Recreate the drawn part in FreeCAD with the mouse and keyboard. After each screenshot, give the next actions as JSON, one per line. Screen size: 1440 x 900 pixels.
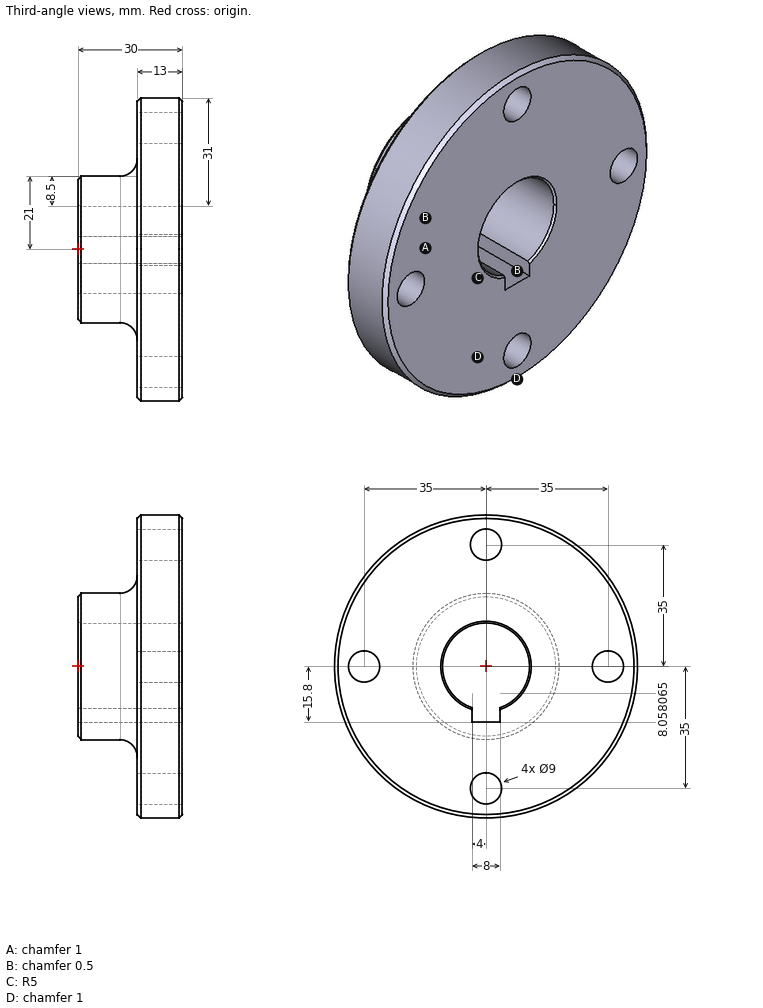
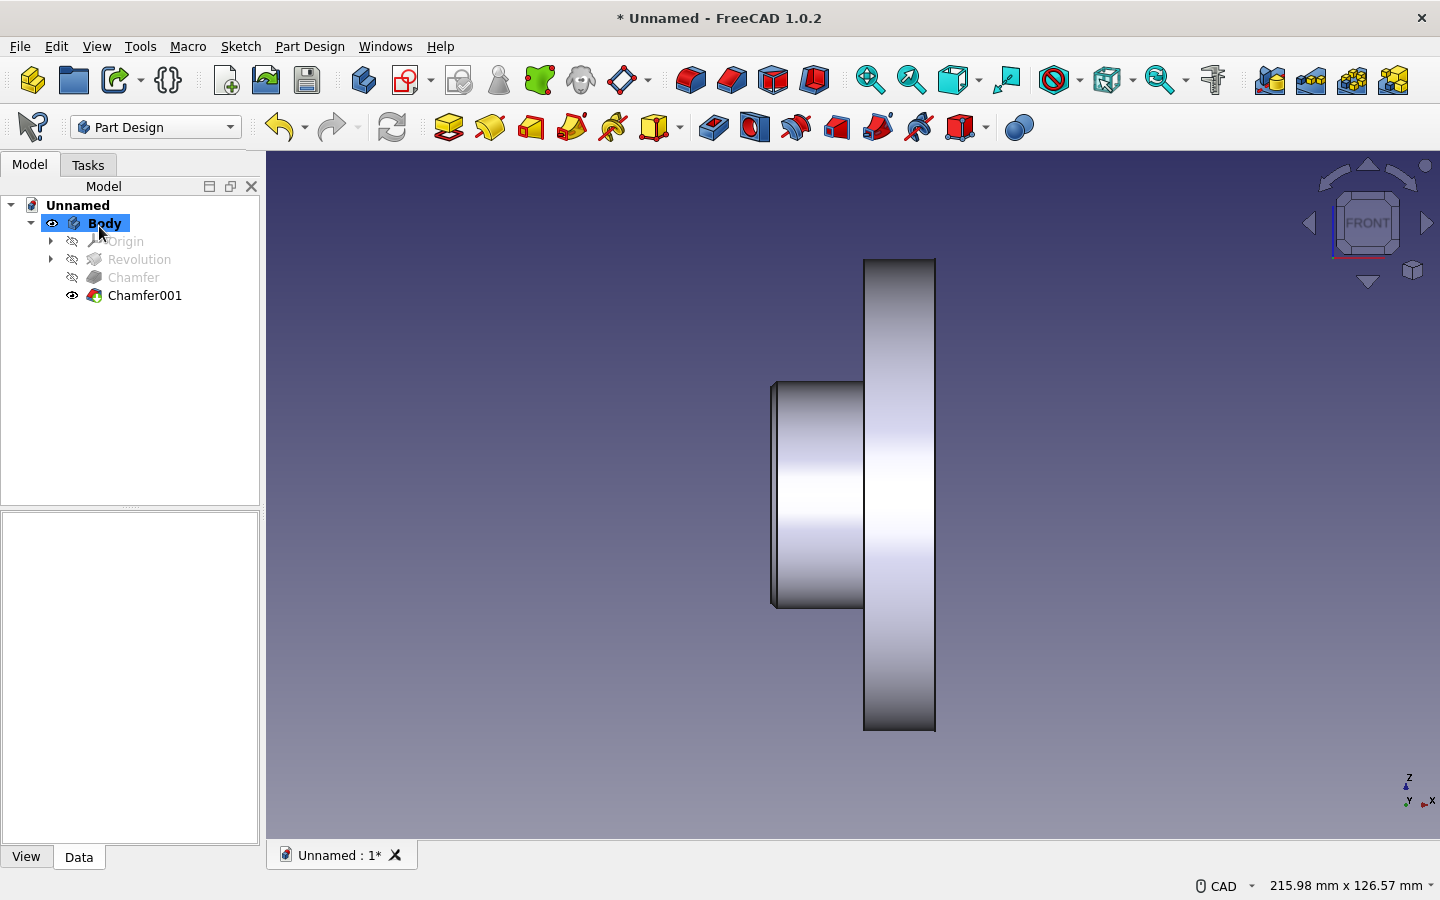
{"action": "key", "text": "3"}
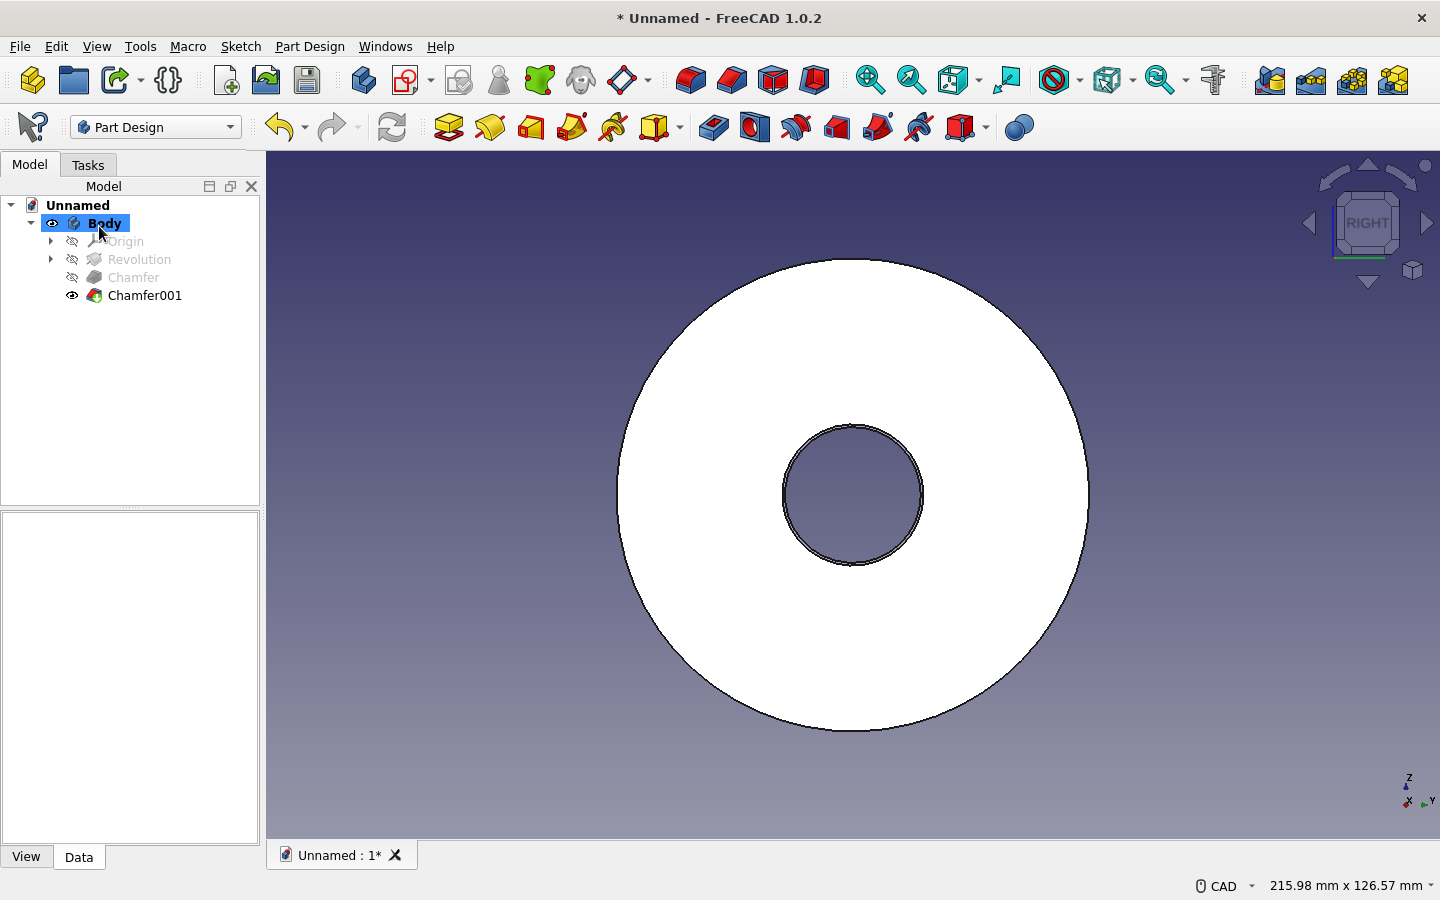
{"action": "key", "text": "5"}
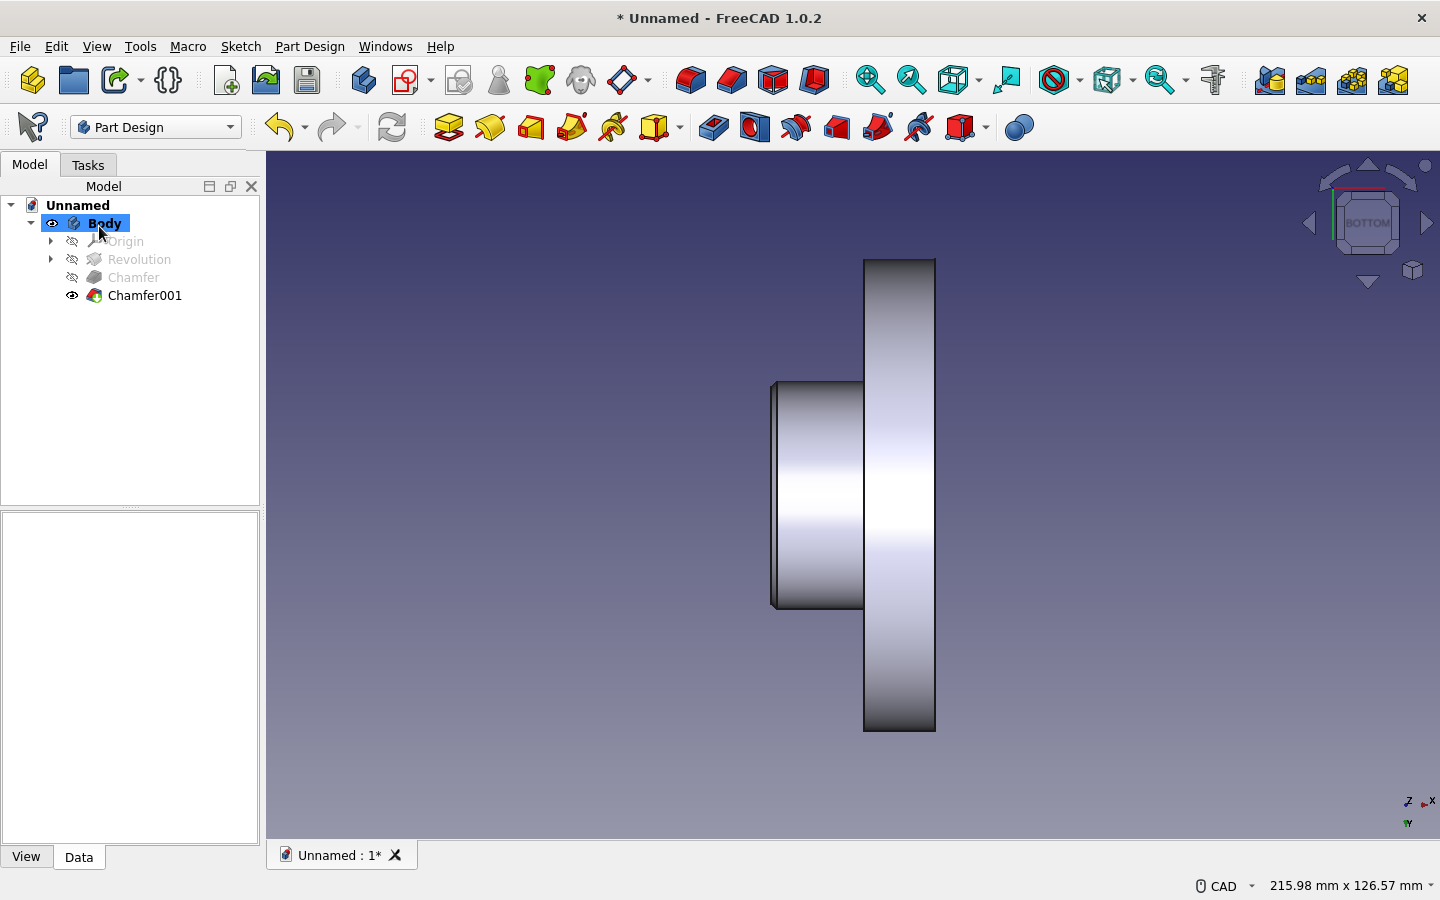
{"action": "key", "text": "4"}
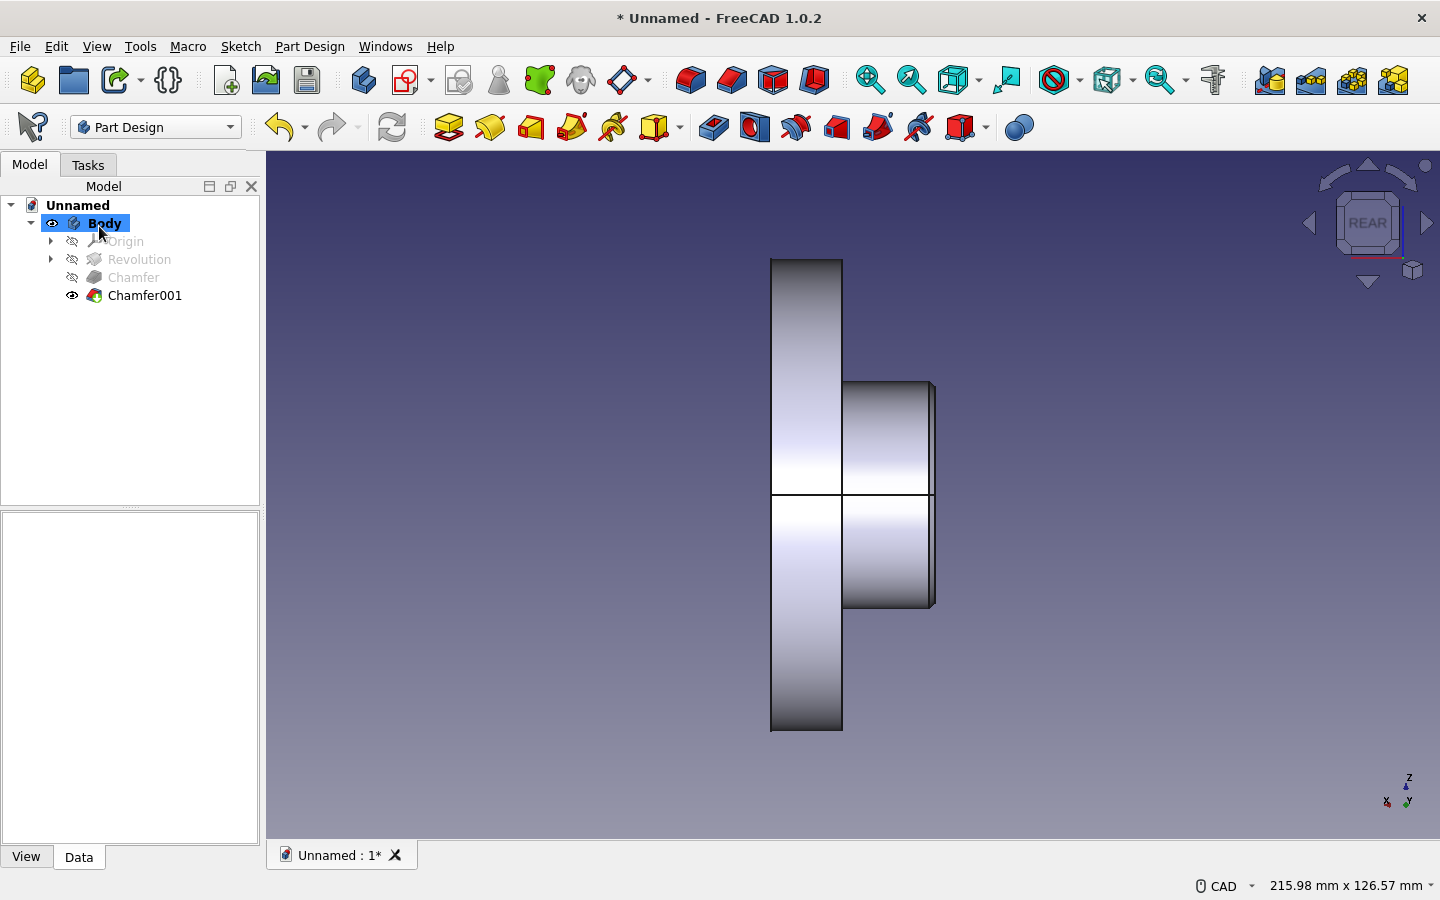
{"action": "key", "text": "6"}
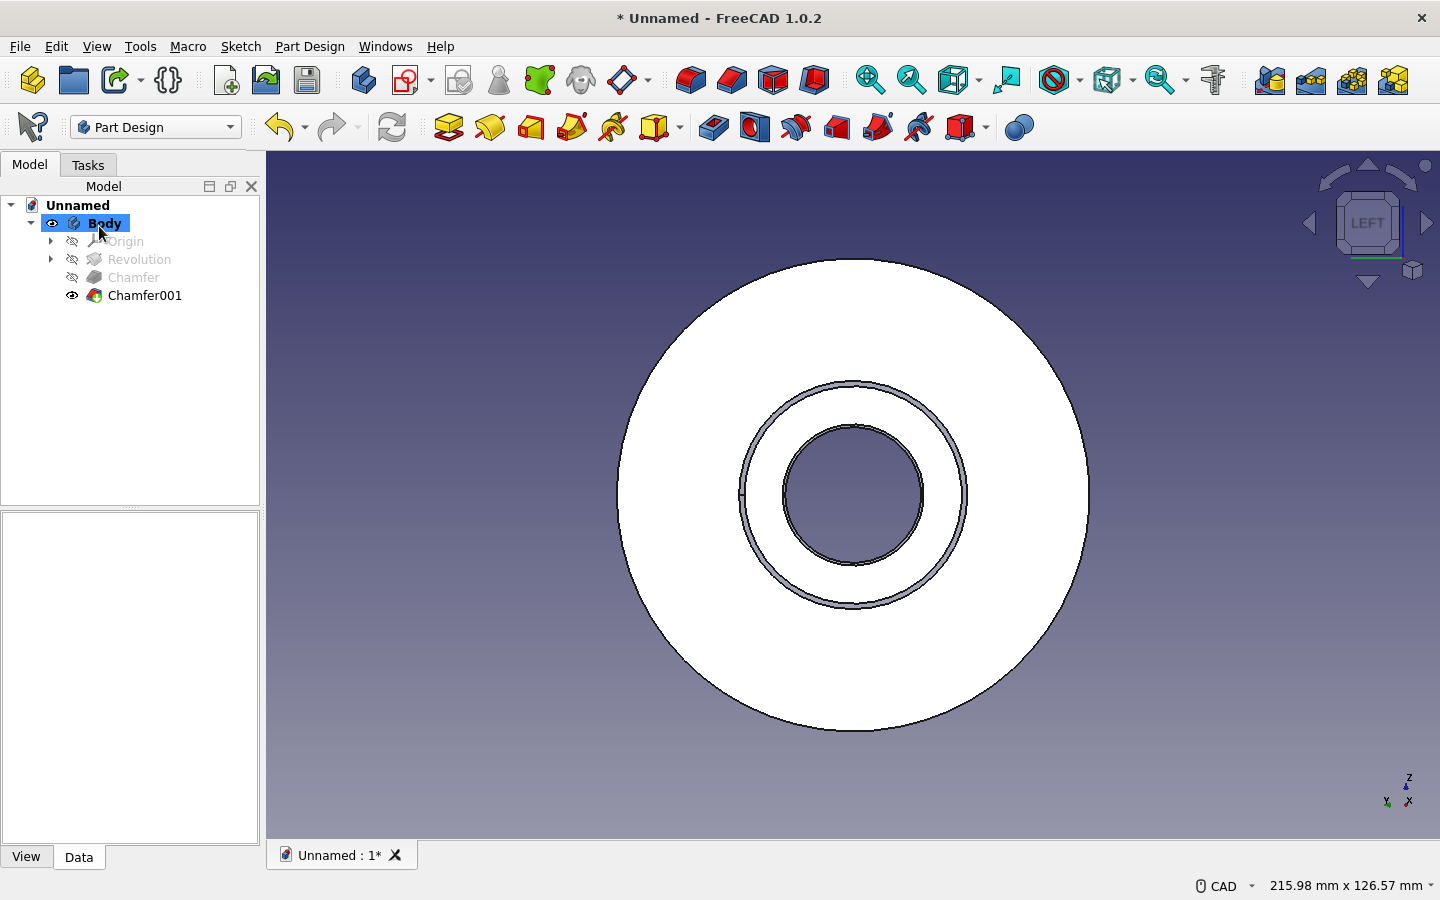
{"action": "key", "text": "v 3"}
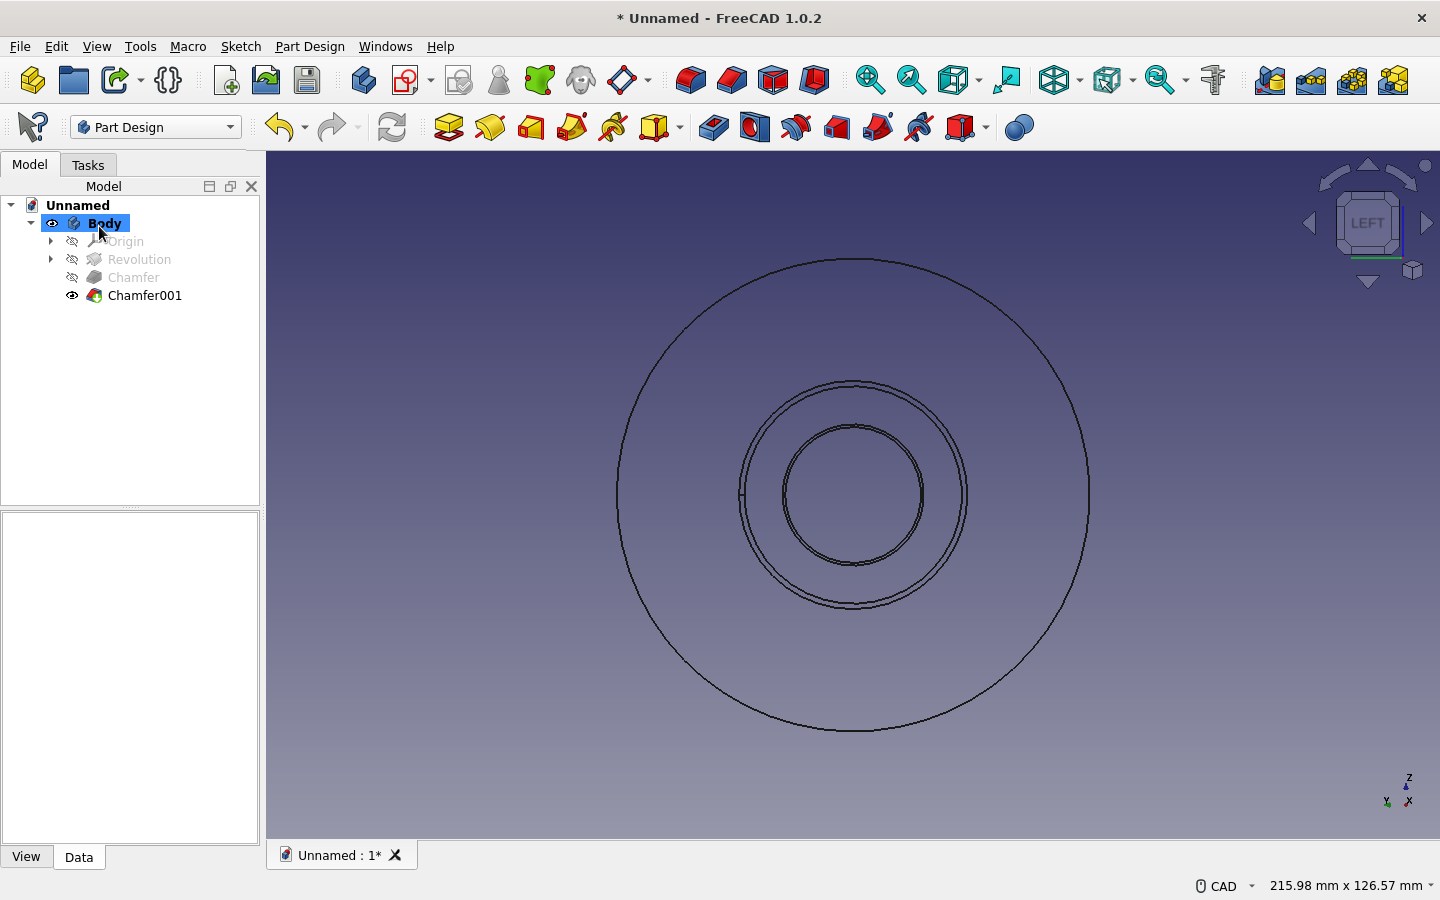
{"action": "key", "text": "0"}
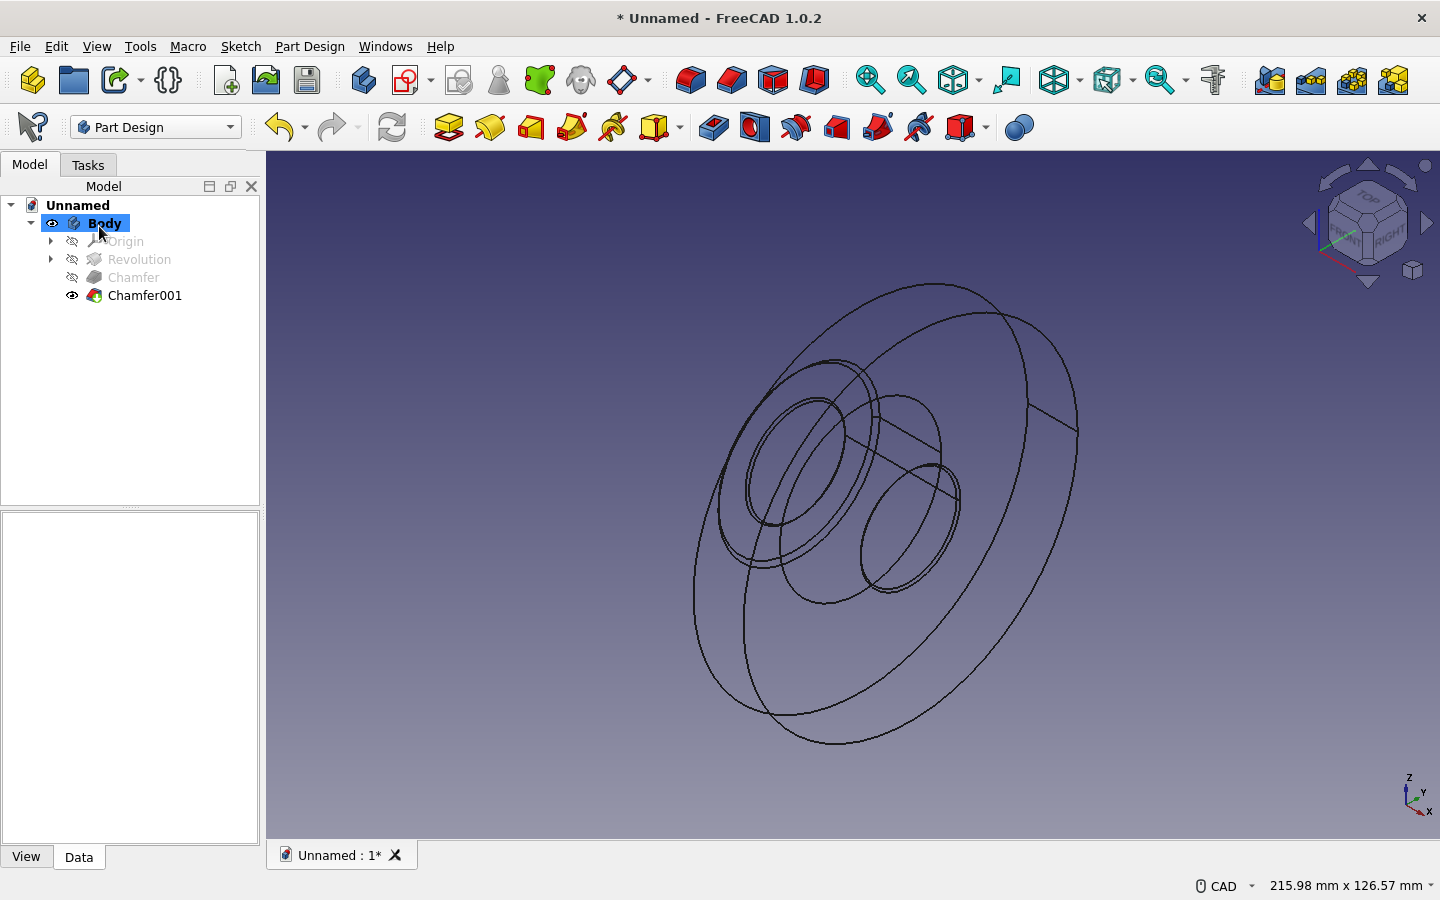
{"action": "left_click", "coordinate": [780, 545]}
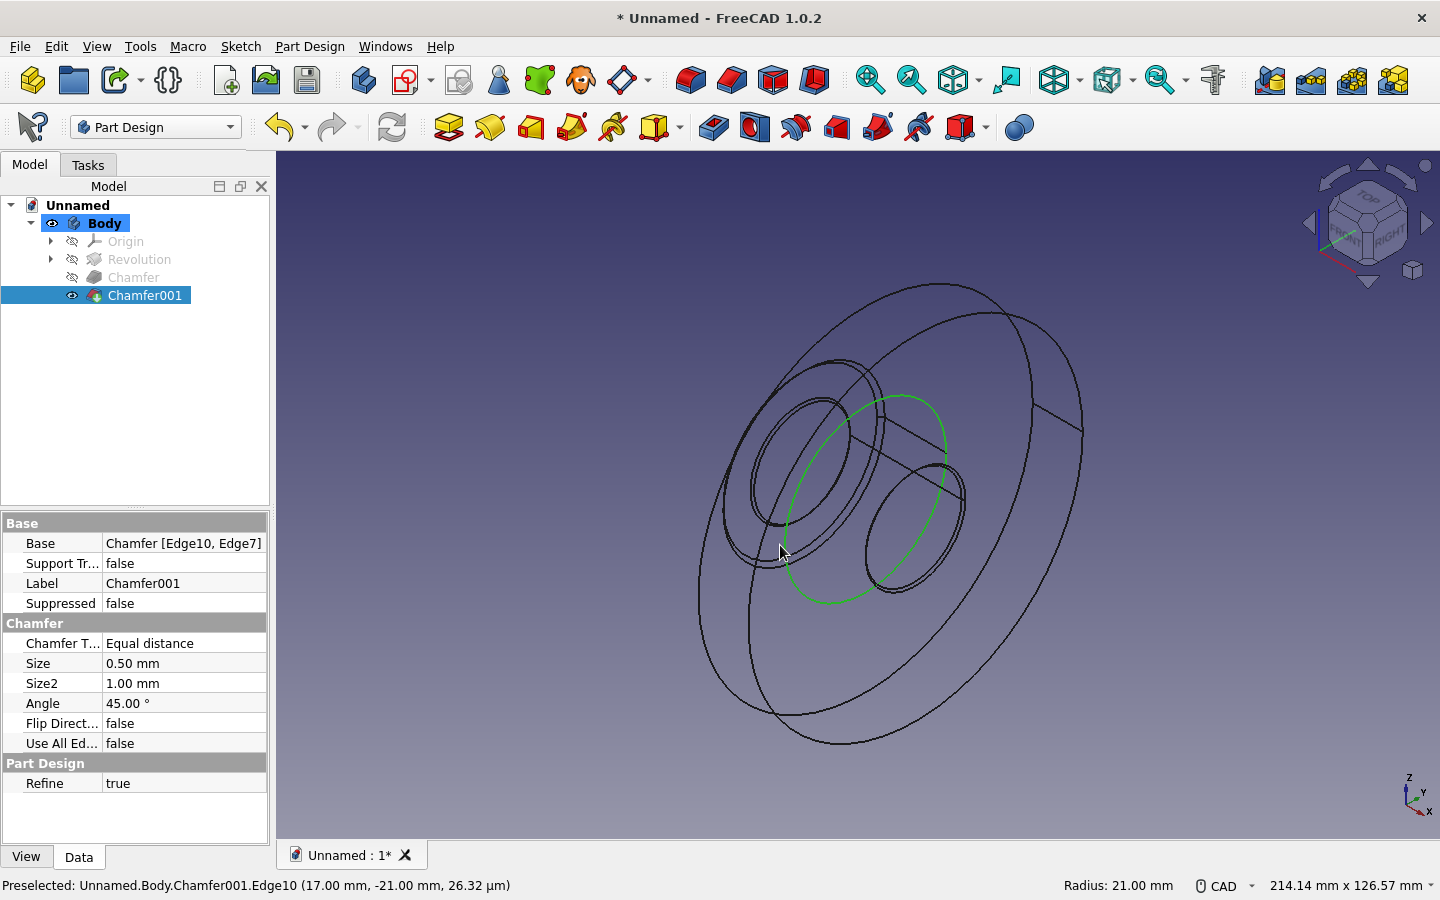
{"action": "key", "text": "v 1"}